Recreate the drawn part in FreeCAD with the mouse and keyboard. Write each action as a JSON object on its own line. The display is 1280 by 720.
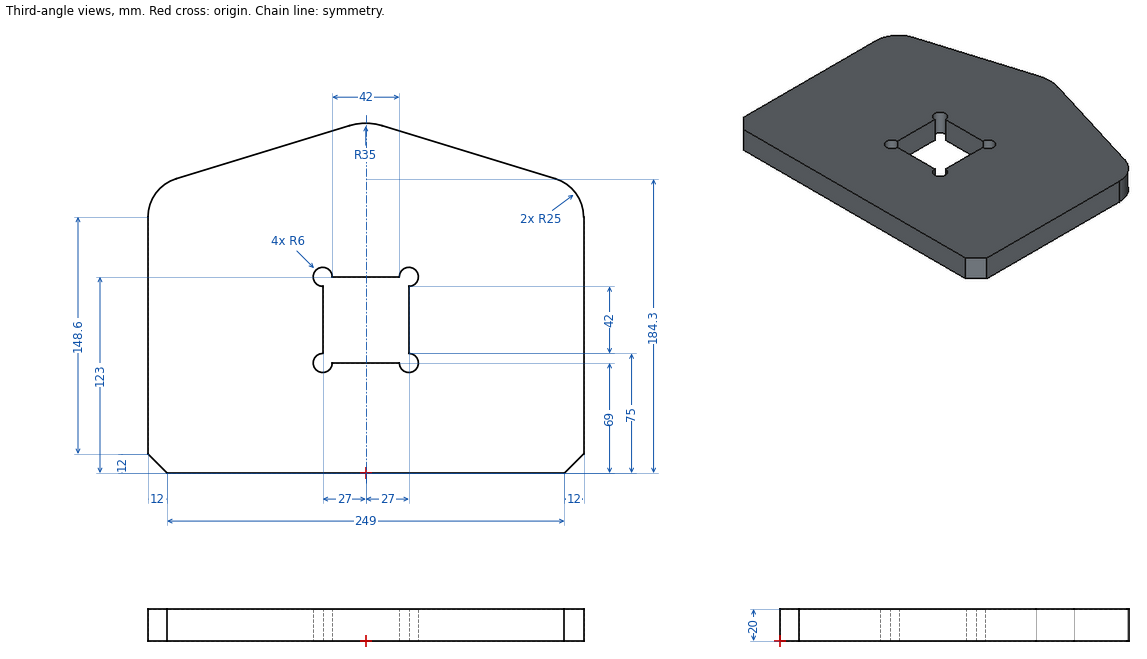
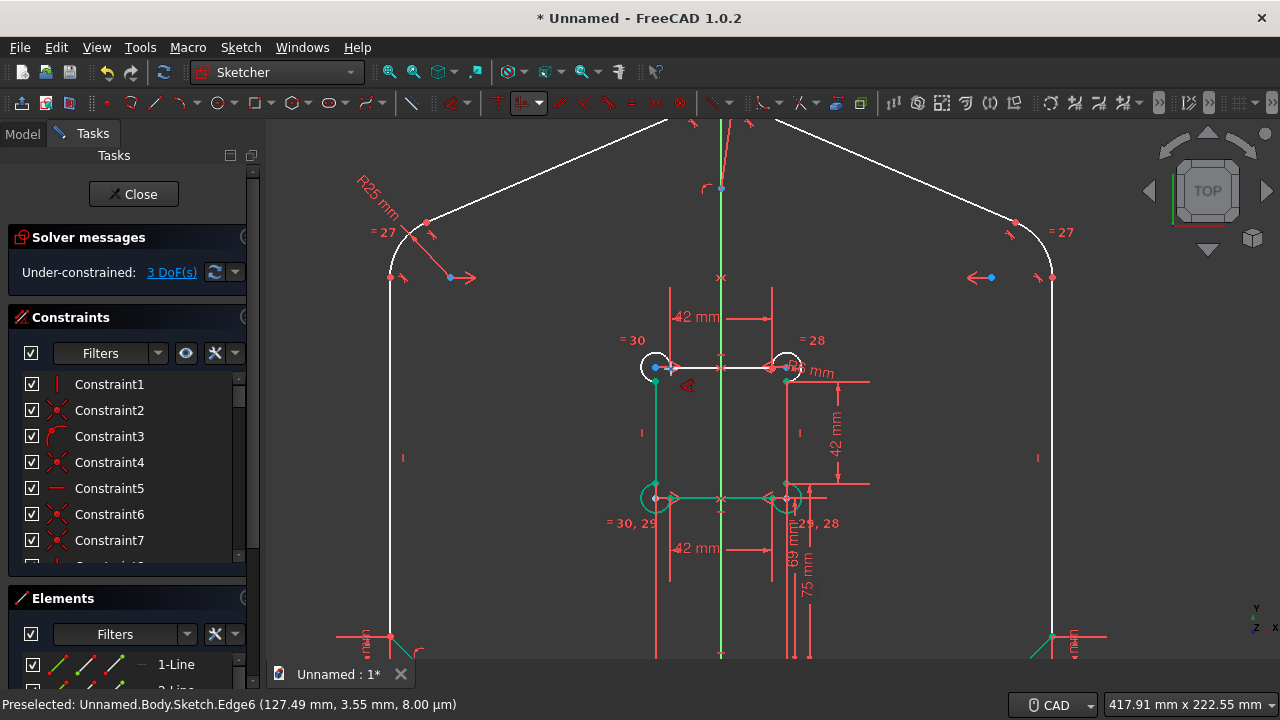
{"action": "left_click", "coordinate": [670, 368]}
{"action": "left_click", "coordinate": [636, 439]}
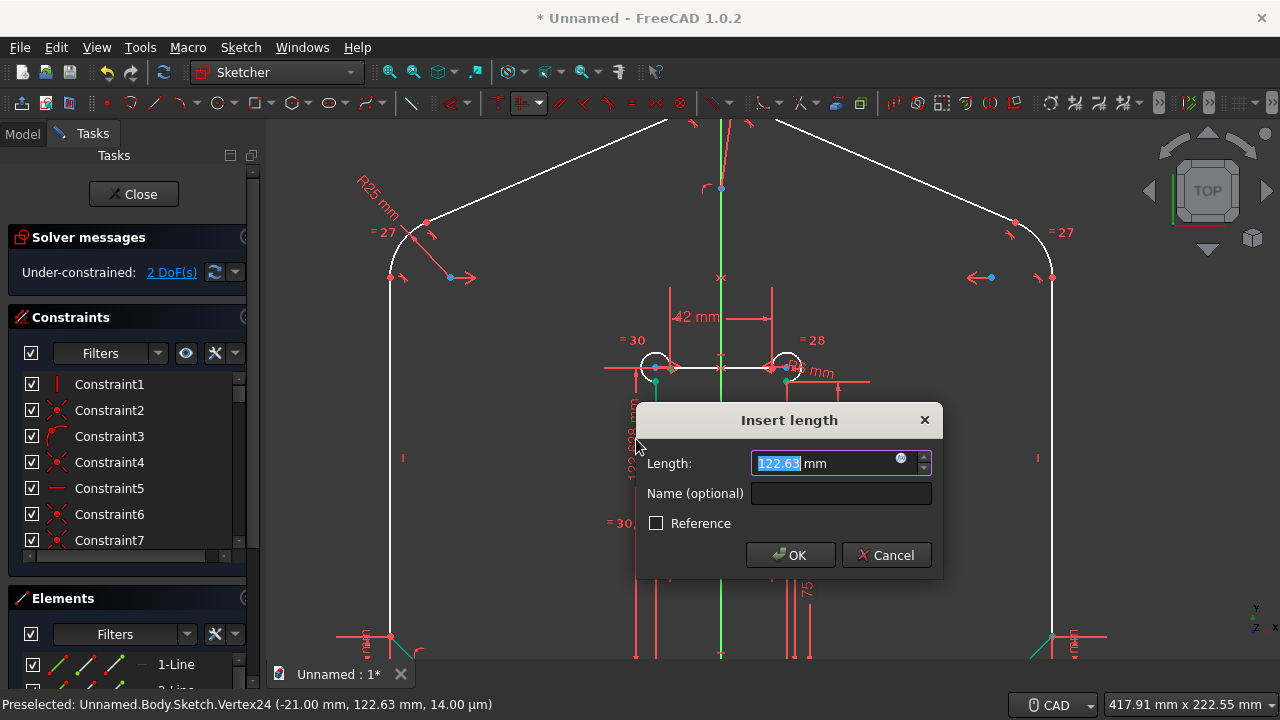
{"action": "type", "text": "123"}
{"action": "key", "text": "Return"}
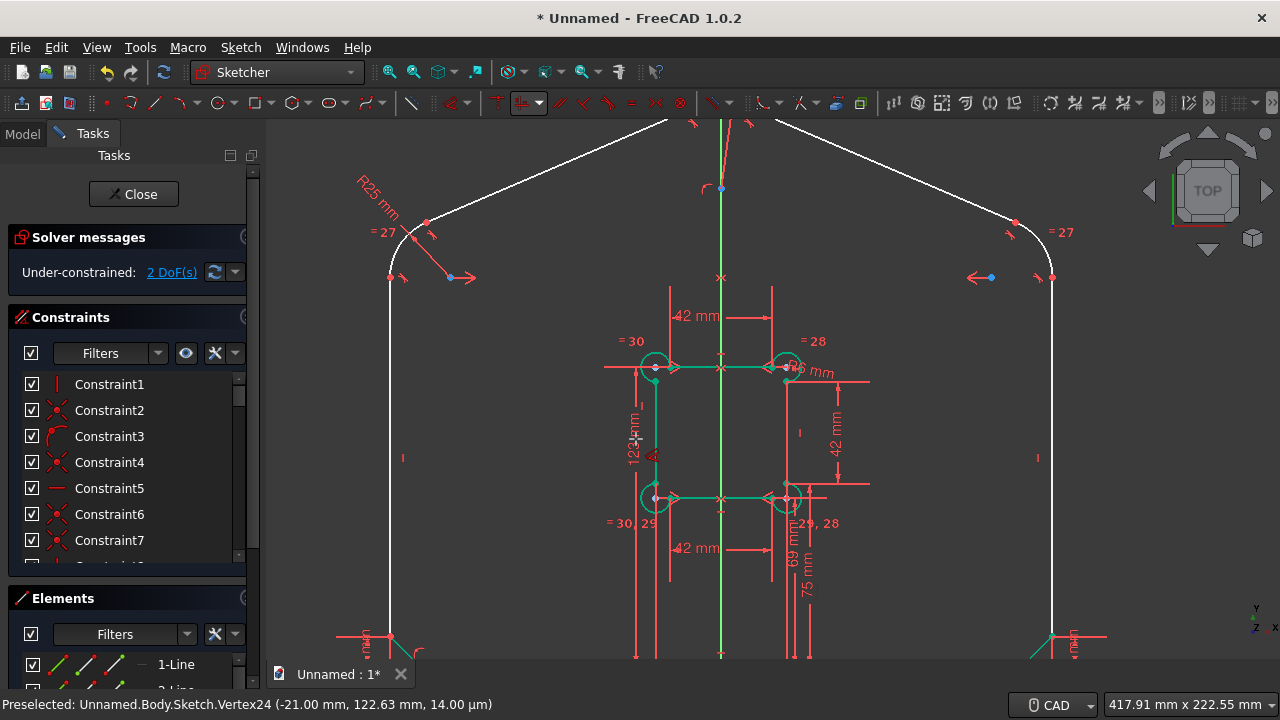
{"action": "left_click", "coordinate": [390, 386]}
{"action": "left_click", "coordinate": [356, 454]}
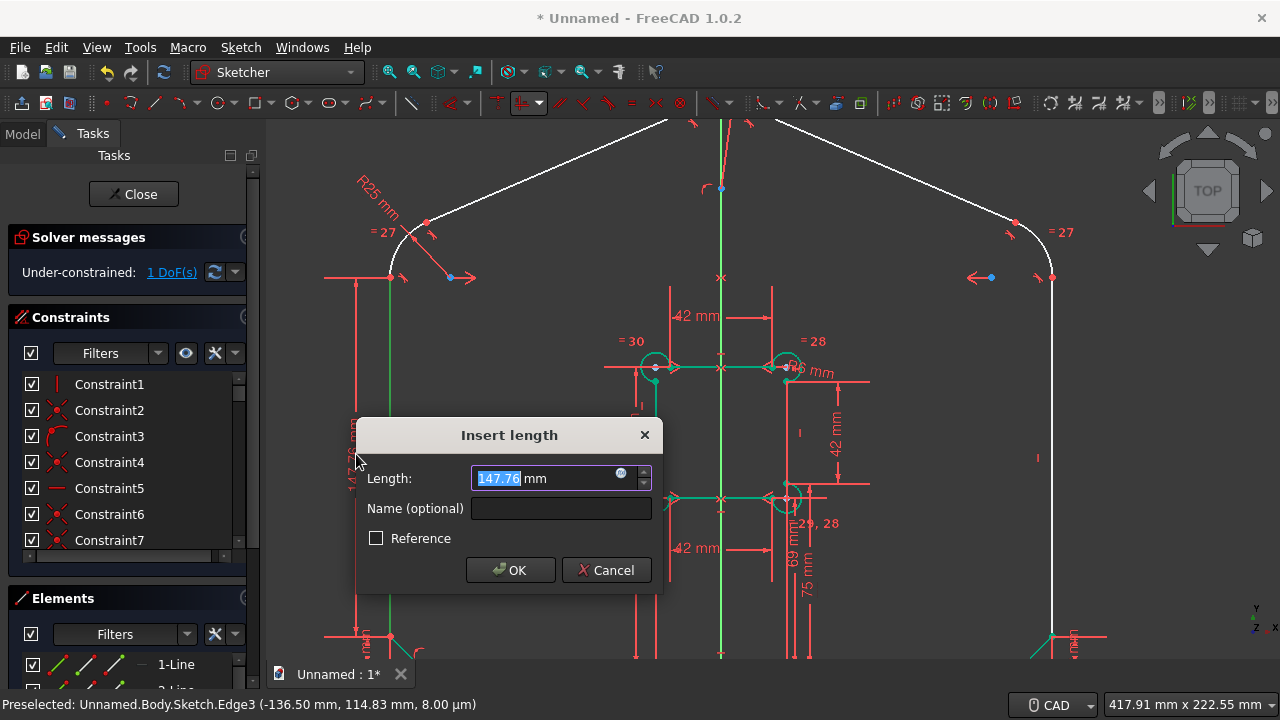
{"action": "type", "text": "148.6"}
{"action": "key", "text": "Return"}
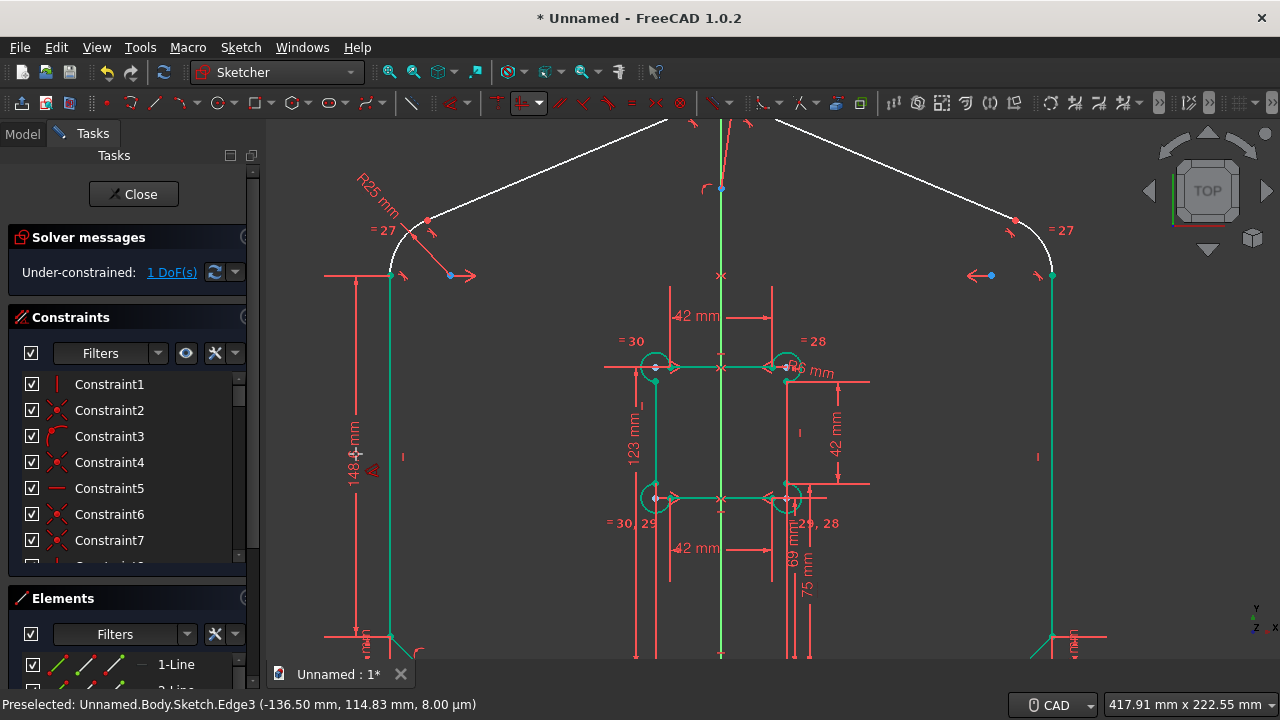
{"action": "left_click", "coordinate": [721, 189]}
{"action": "left_click", "coordinate": [755, 410]}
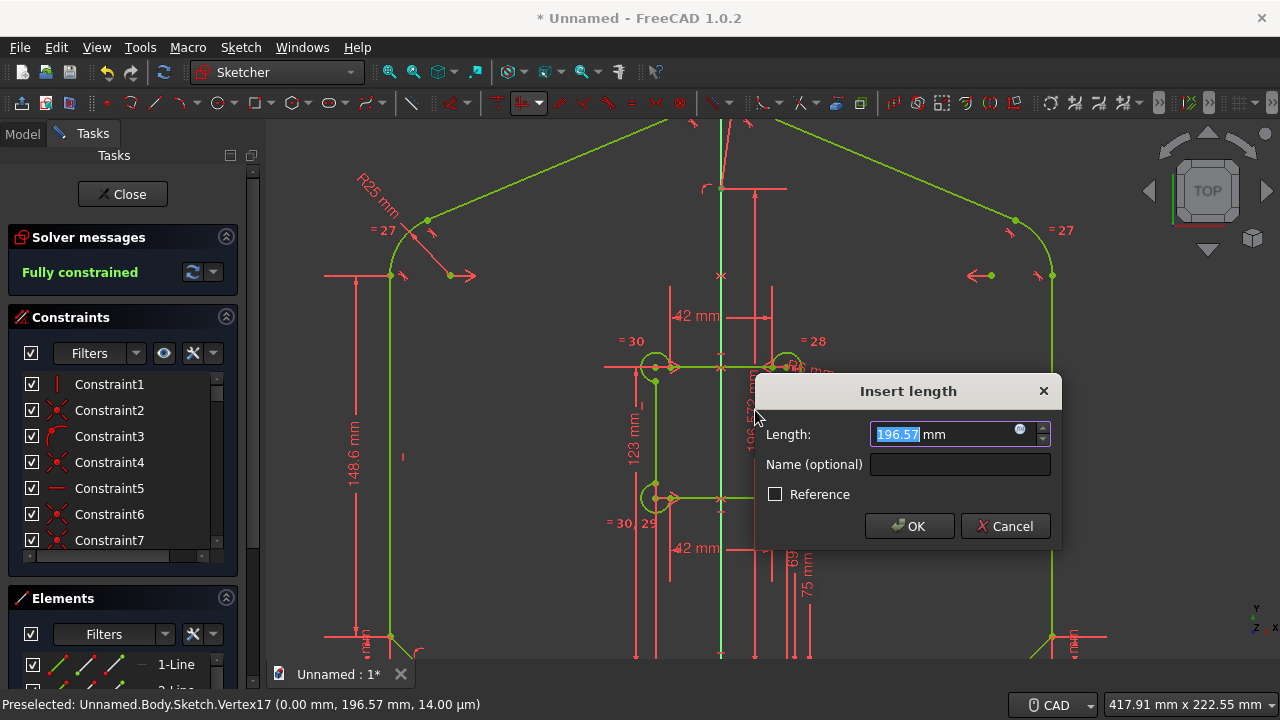
{"action": "type", "text": "184.3"}
{"action": "key", "text": "Return"}
{"action": "key", "text": "Escape"}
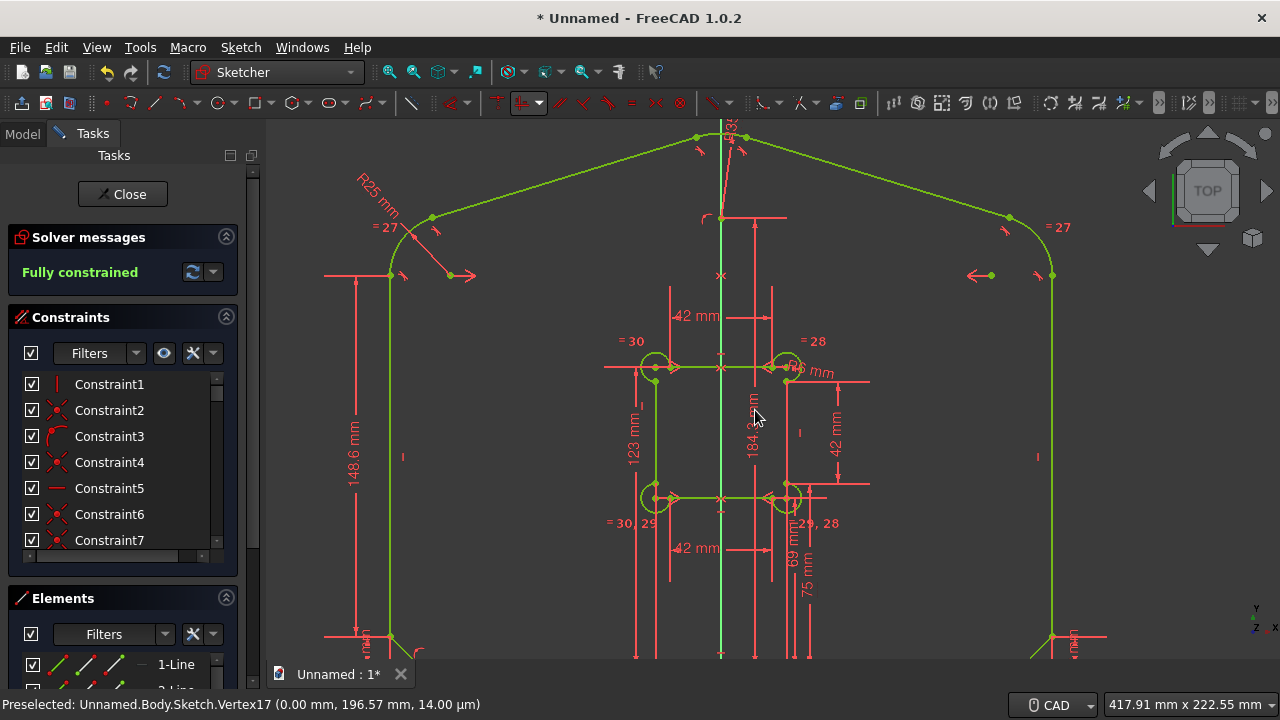
{"action": "left_click", "coordinate": [123, 194]}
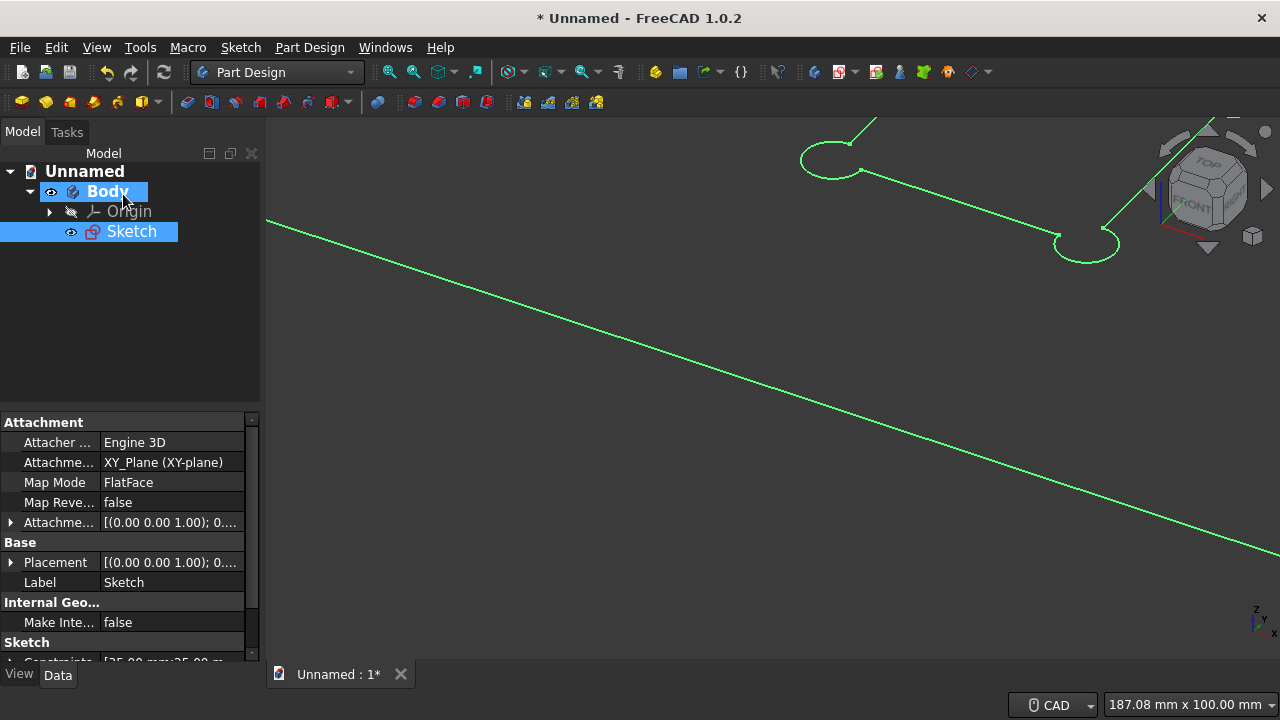
{"action": "left_click", "coordinate": [22, 102]}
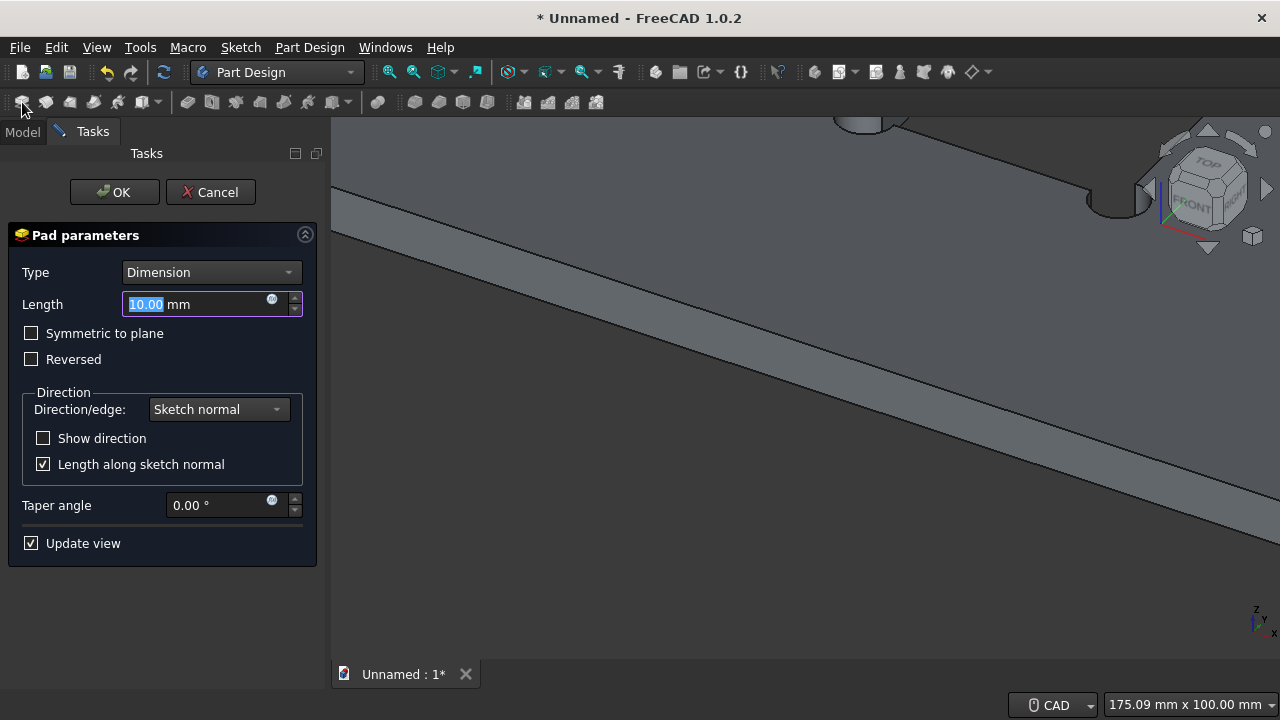
{"action": "type", "text": "20"}
{"action": "key", "text": "Tab"}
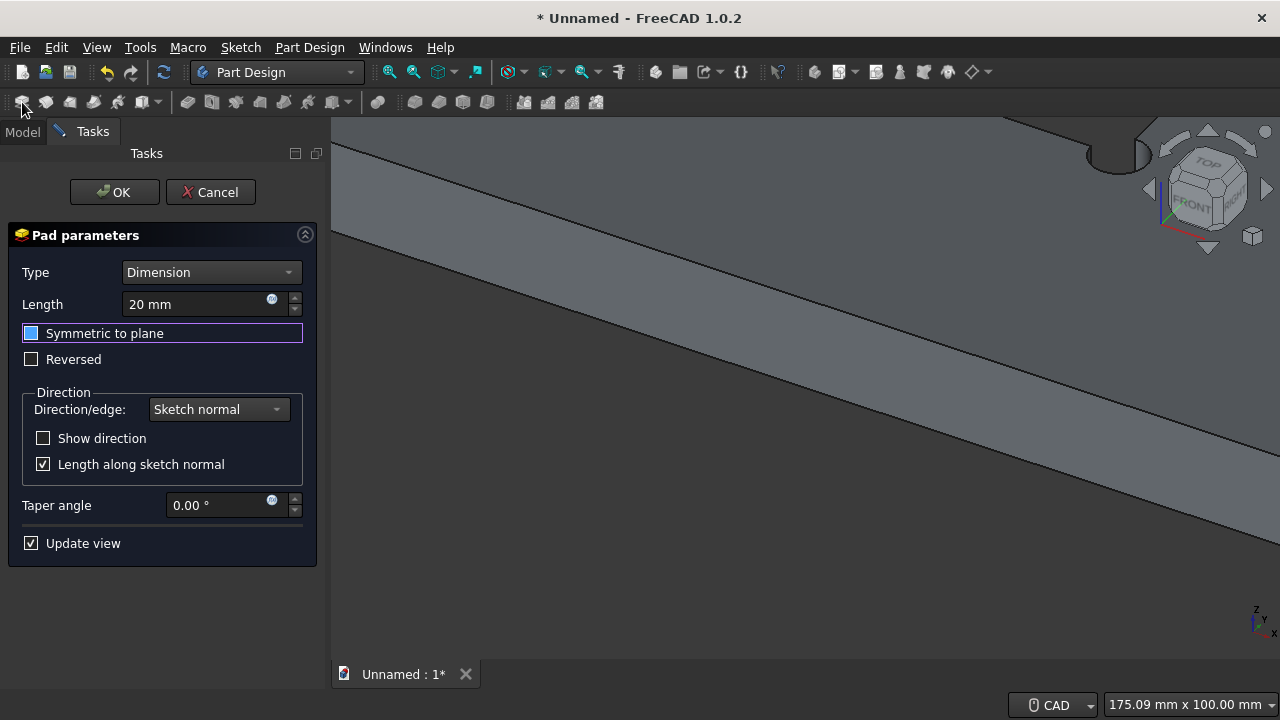
{"action": "left_click", "coordinate": [115, 192]}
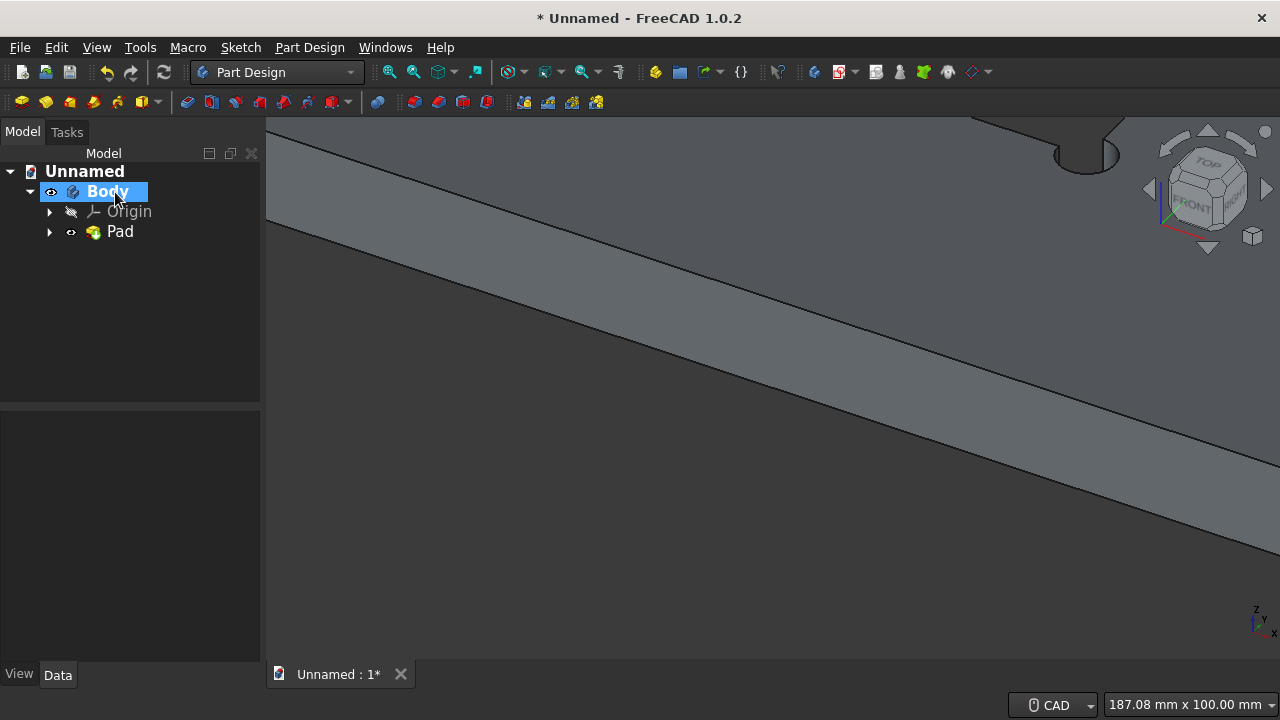
{"action": "key", "text": "0"}